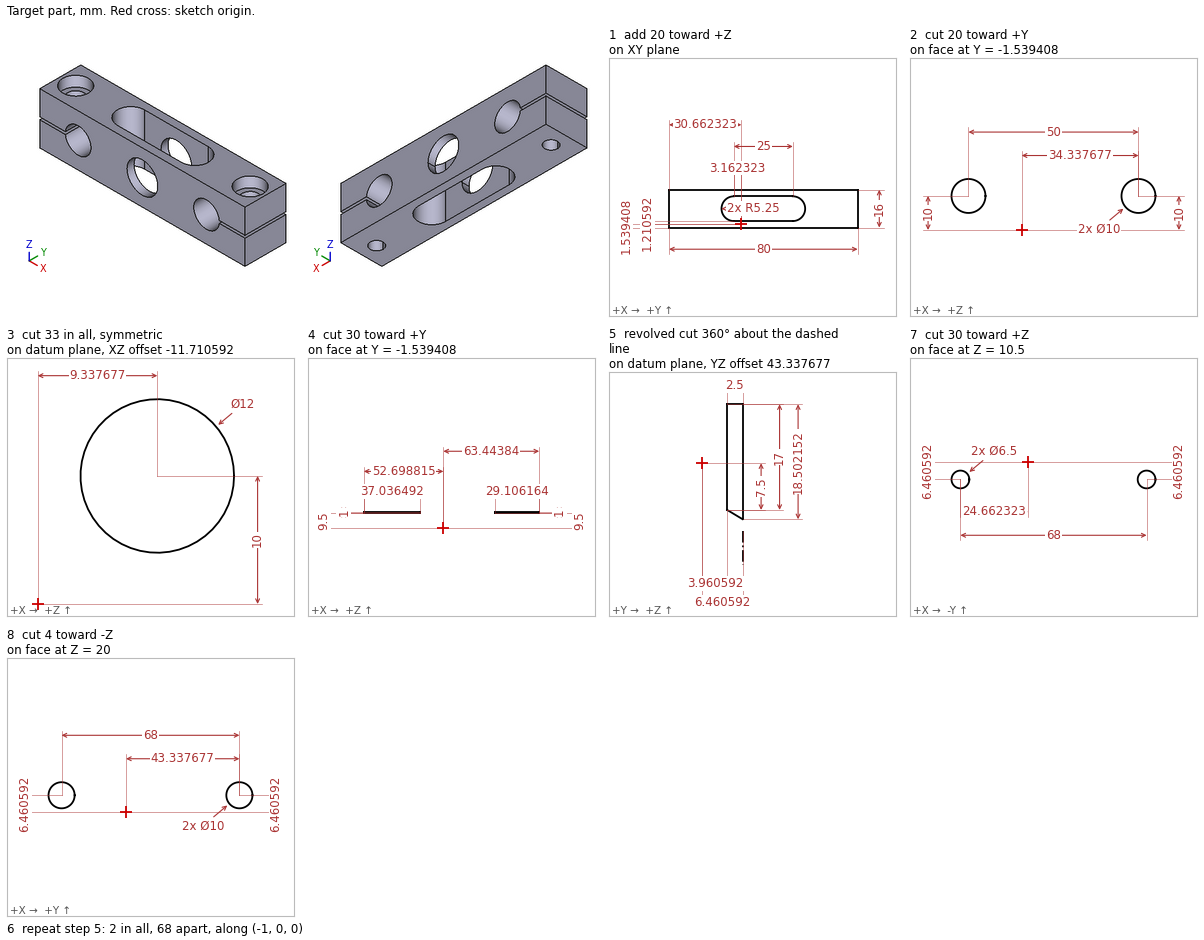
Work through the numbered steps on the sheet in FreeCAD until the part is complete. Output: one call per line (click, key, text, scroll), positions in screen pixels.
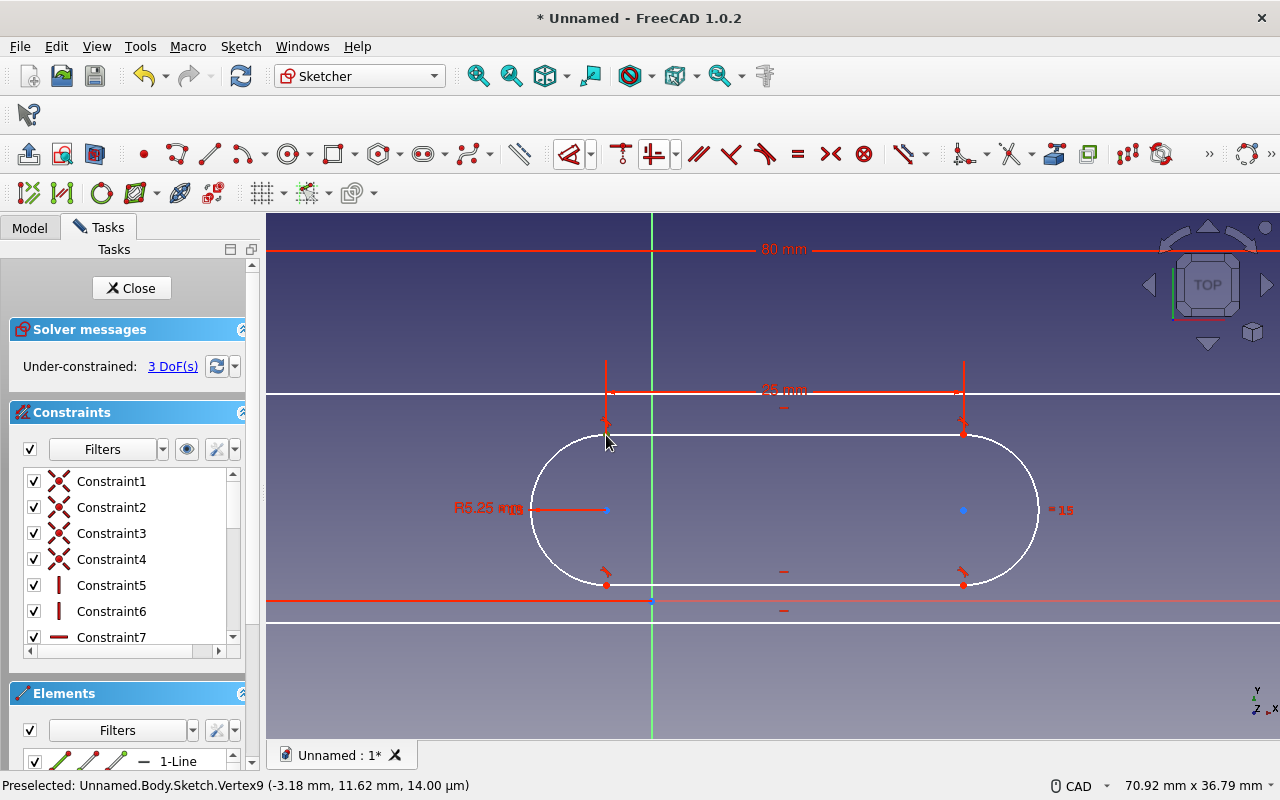
click(590, 154)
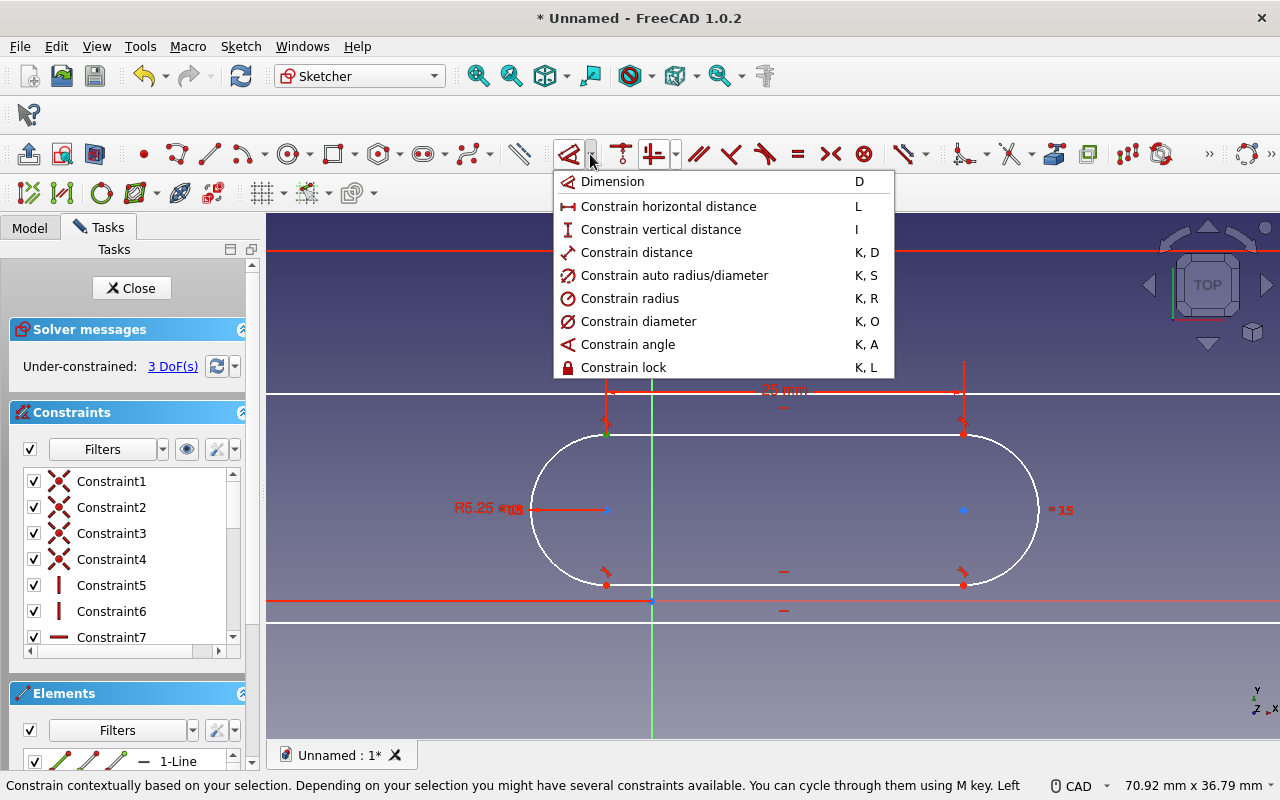
click(724, 206)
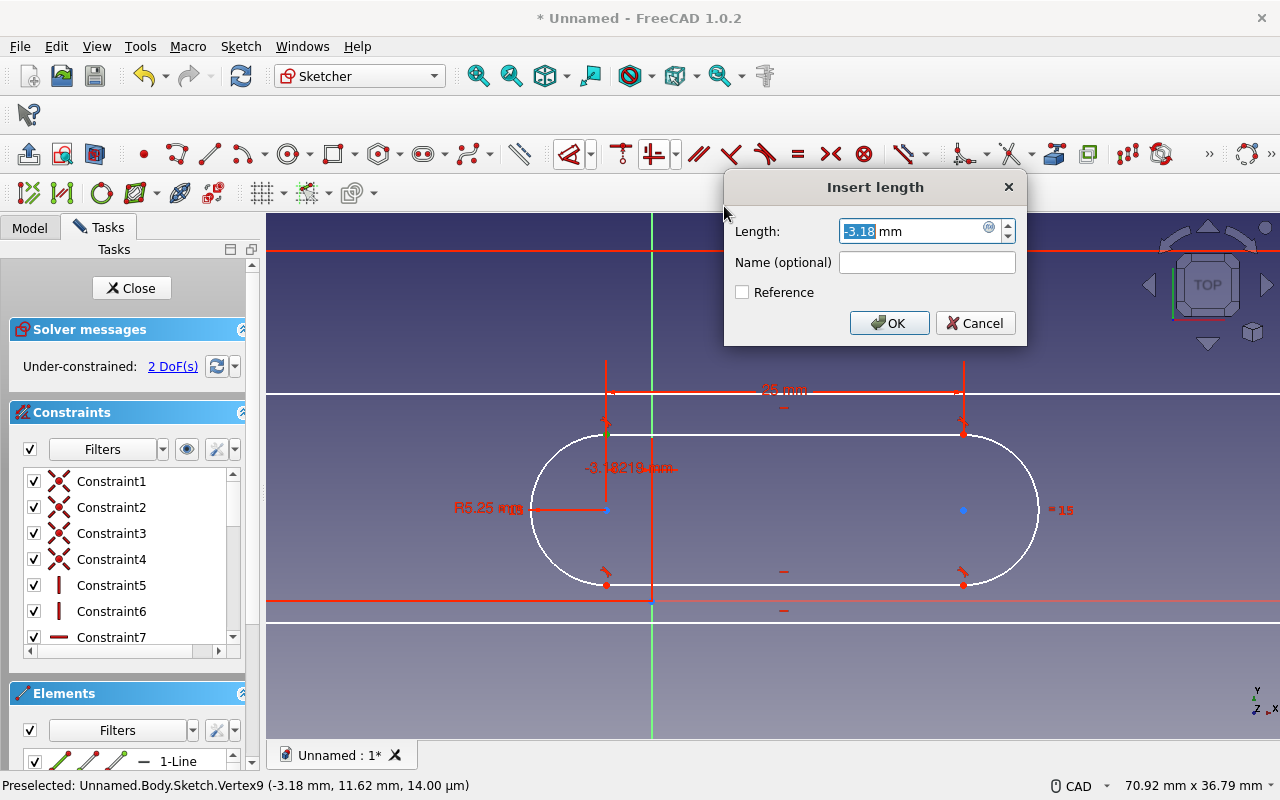
text(-3.162323)
key(Return)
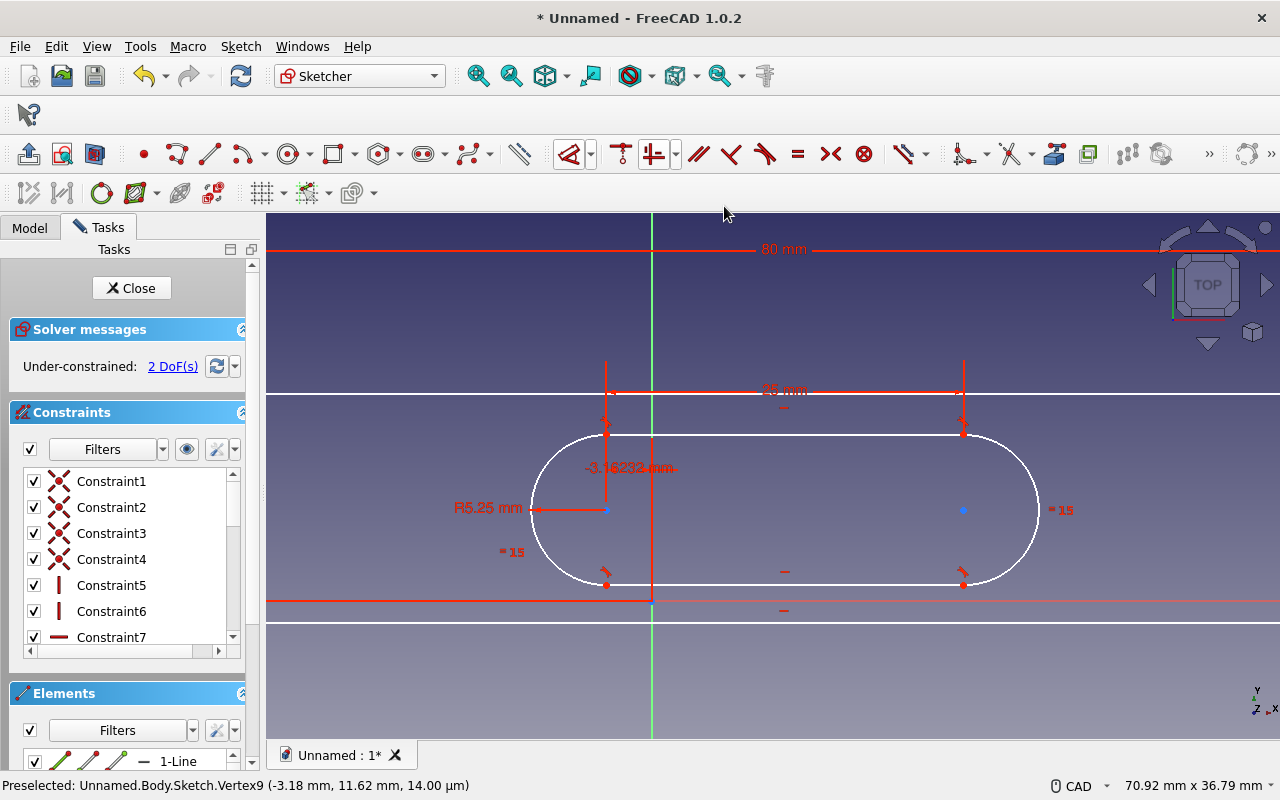
scroll(606, 585, up, 5)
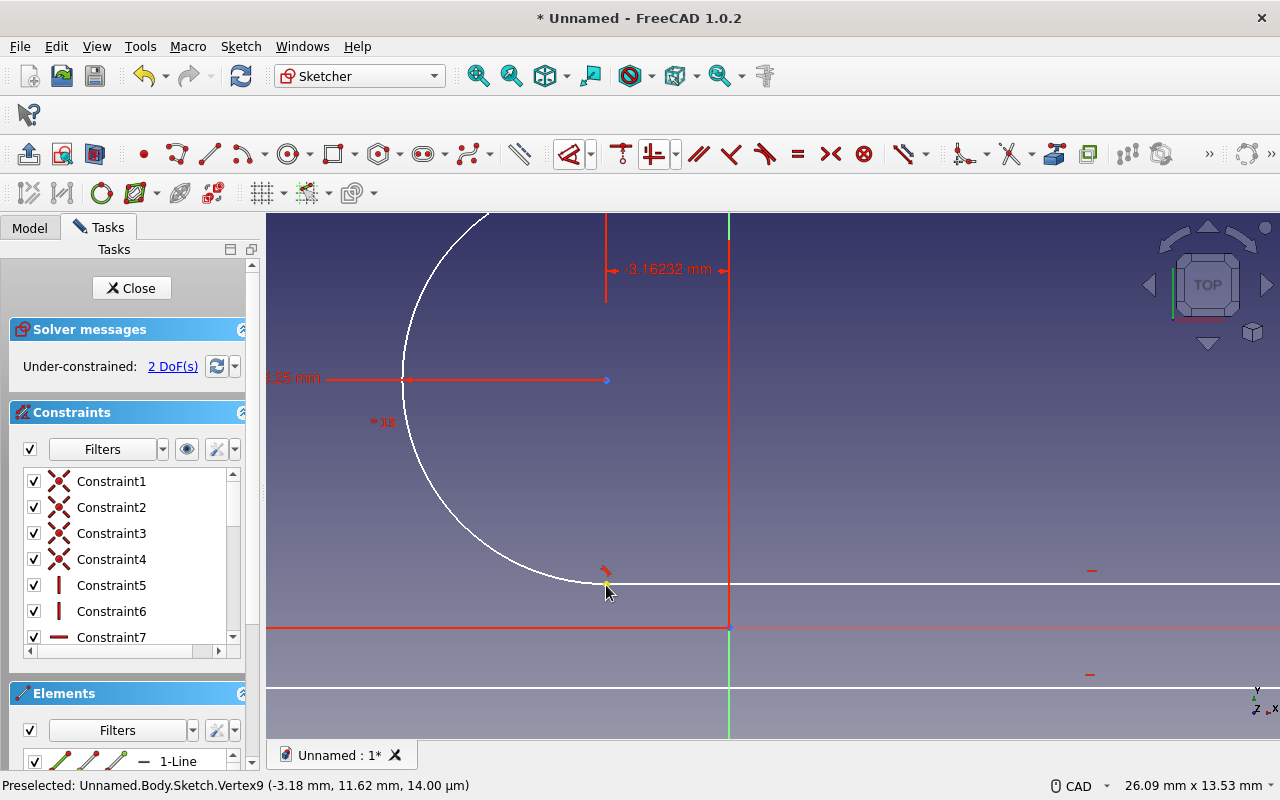
click(606, 584)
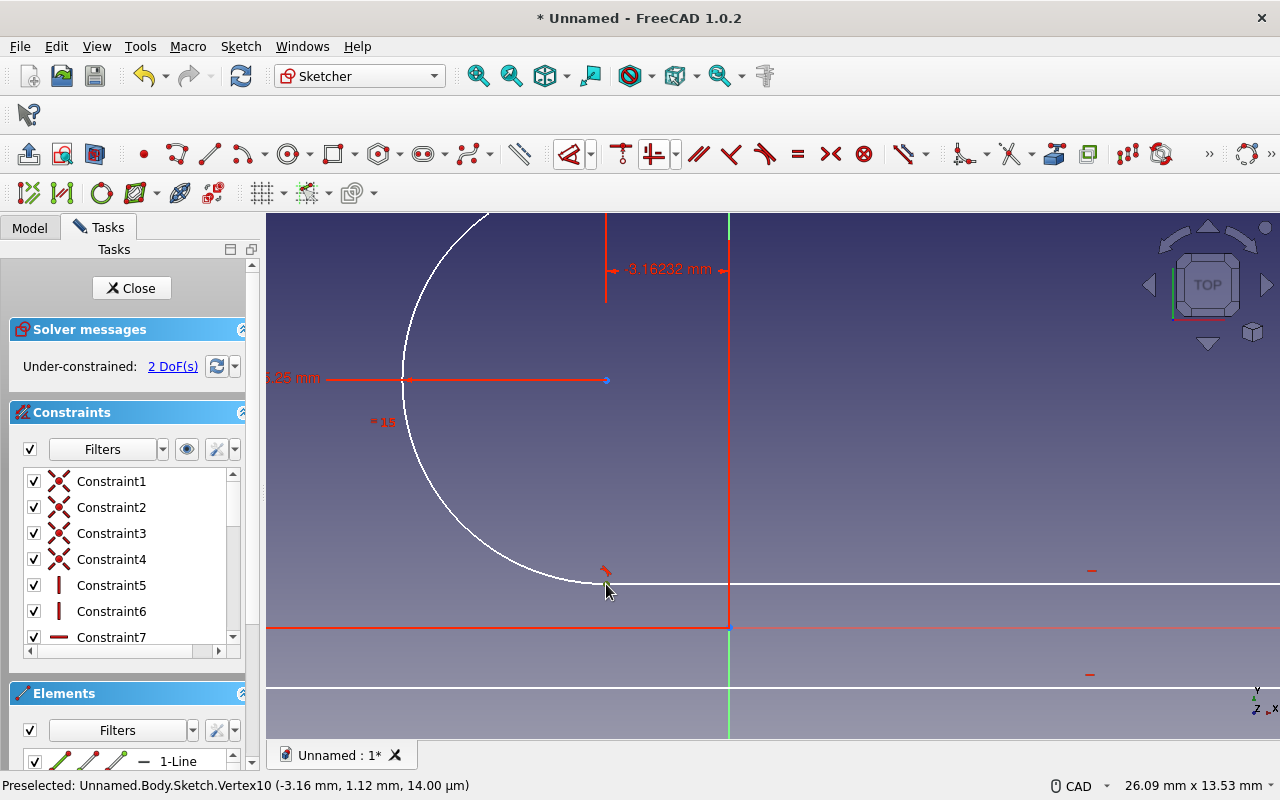
click(590, 154)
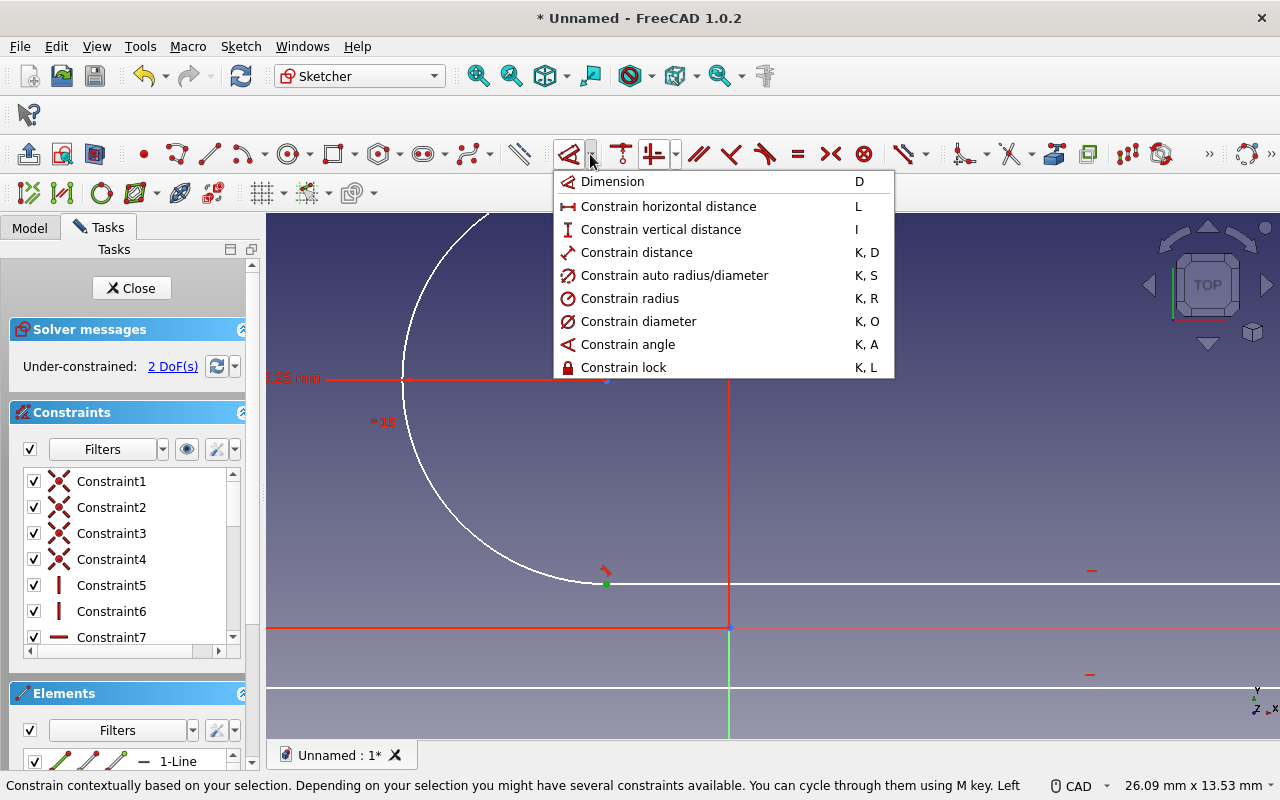
click(724, 230)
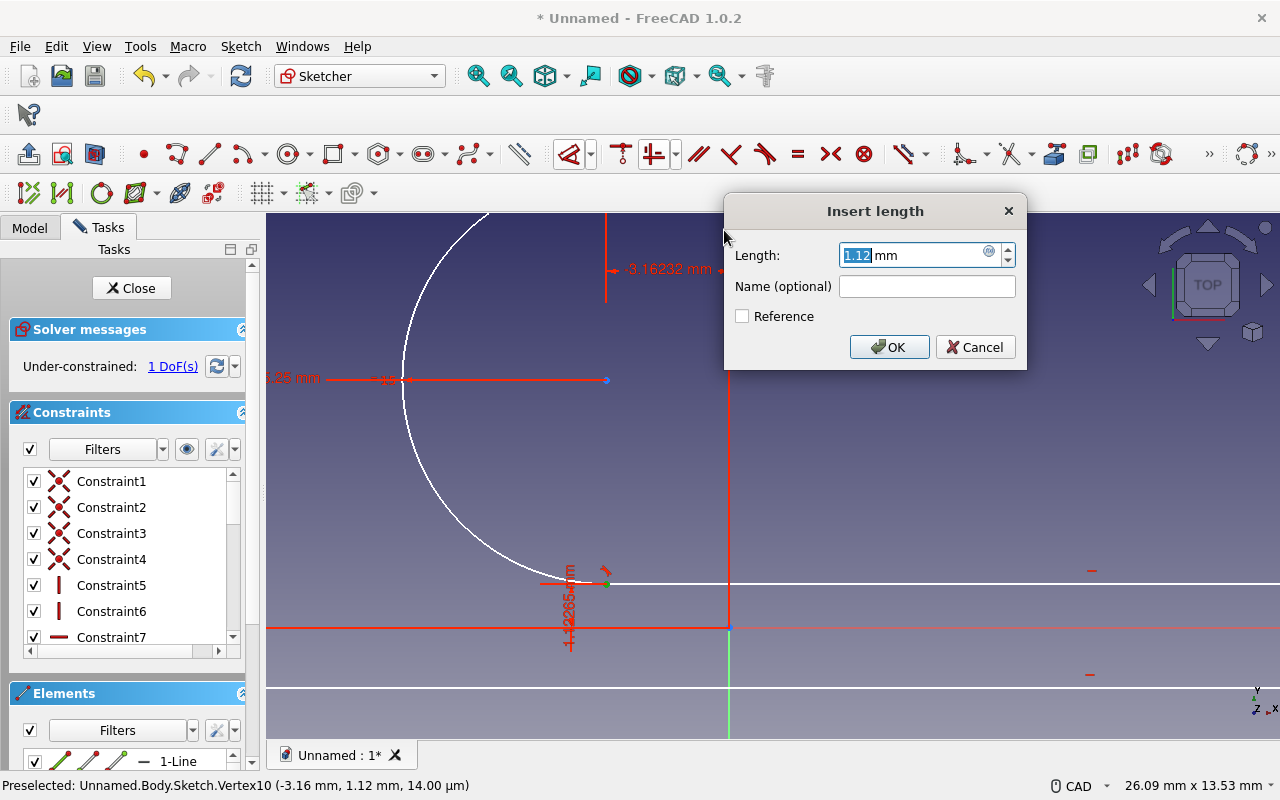
text(1.210592)
key(Return)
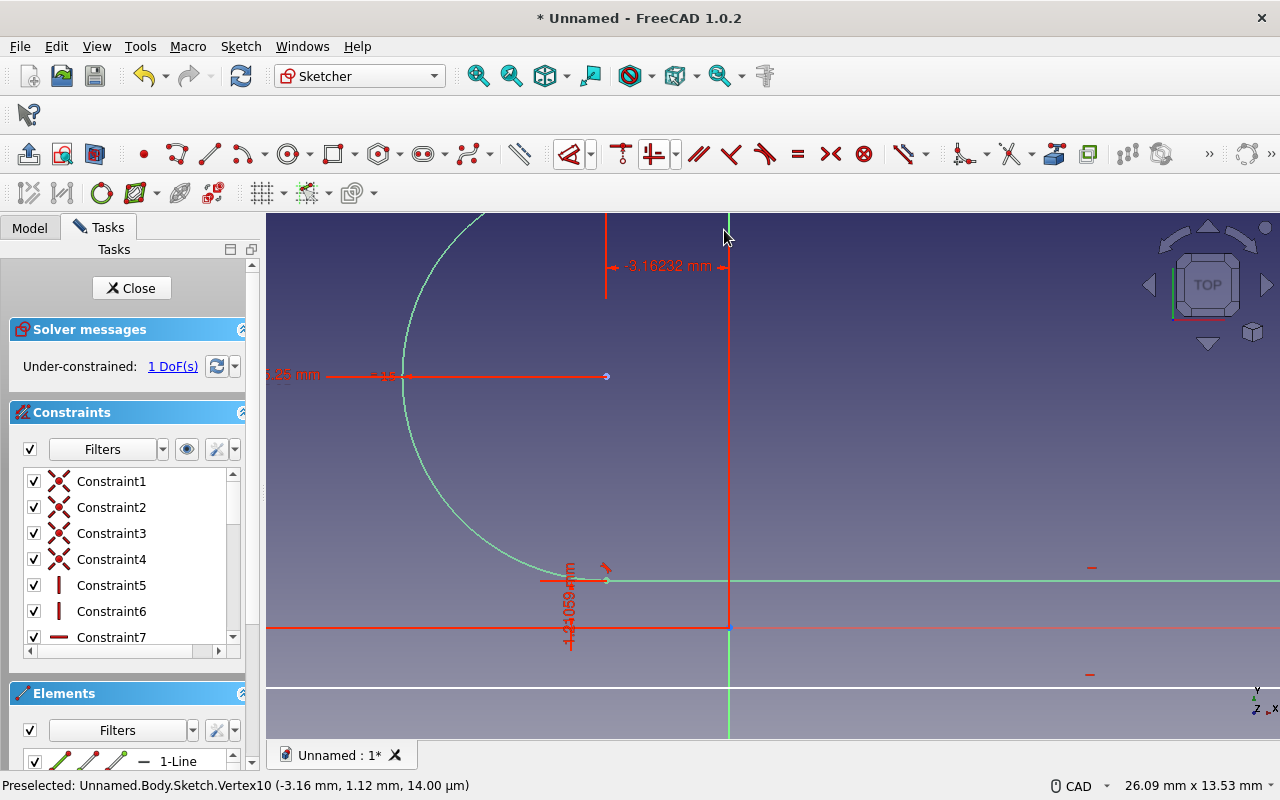
scroll(606, 501, down, 8)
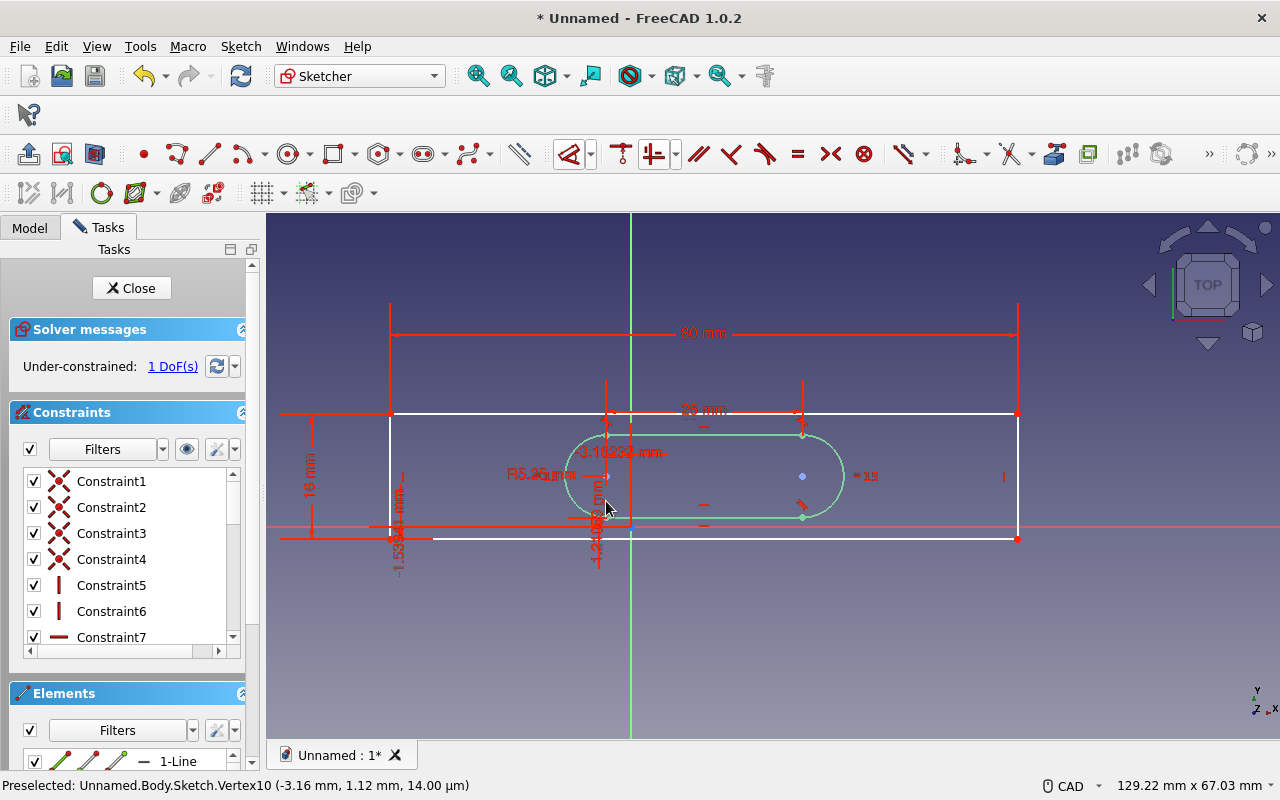
click(390, 414)